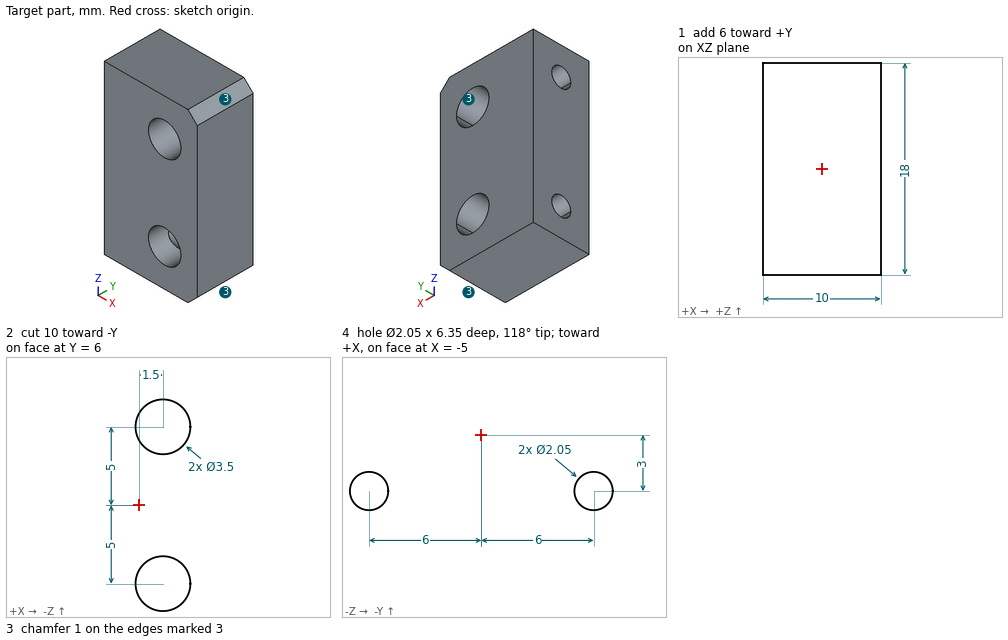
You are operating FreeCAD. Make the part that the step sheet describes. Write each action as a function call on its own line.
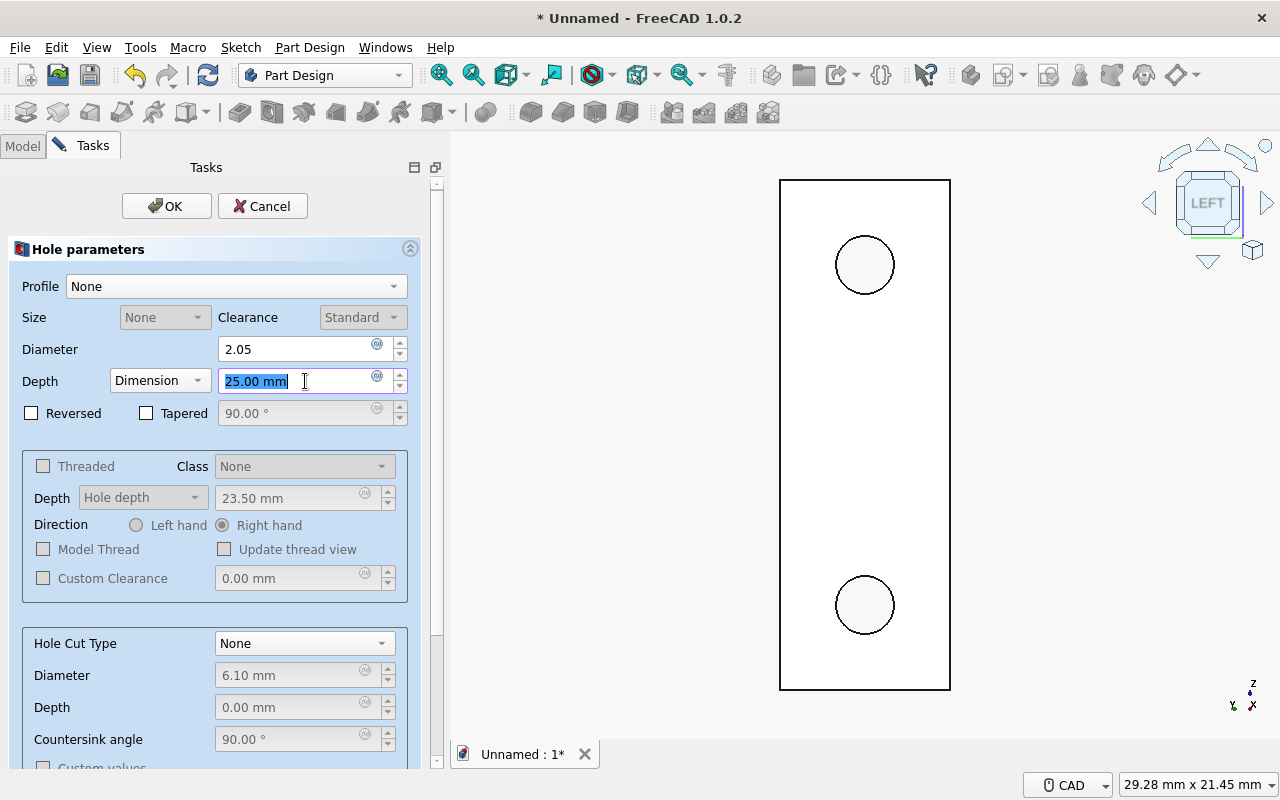
text(6.35)
key(Tab)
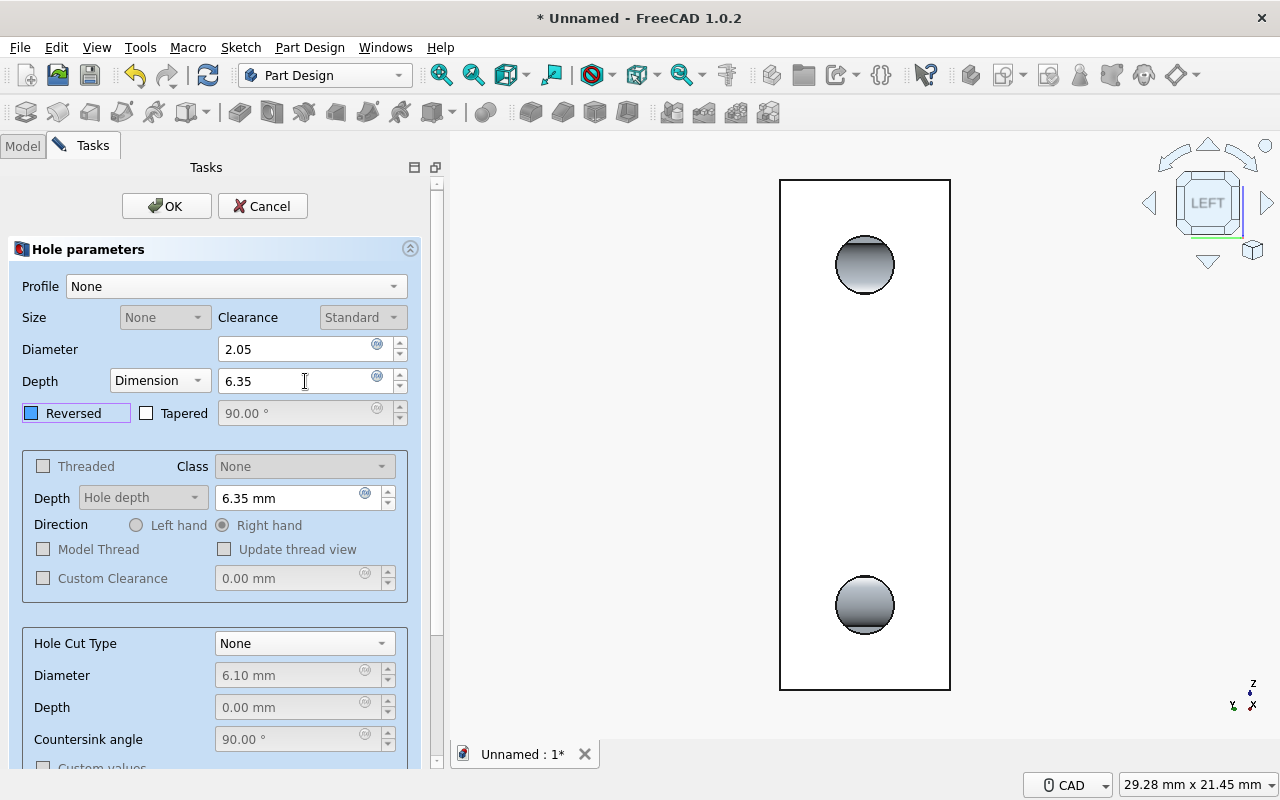
click(167, 206)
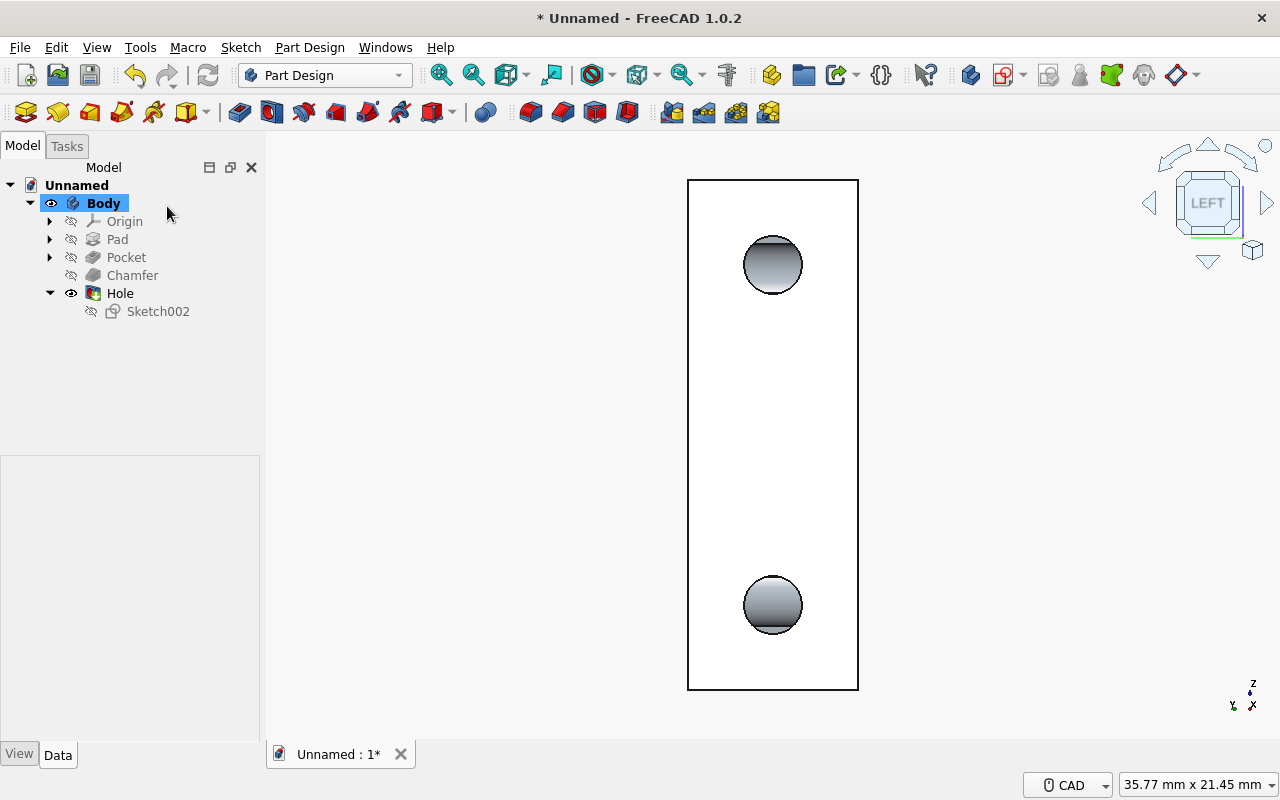
key(0)